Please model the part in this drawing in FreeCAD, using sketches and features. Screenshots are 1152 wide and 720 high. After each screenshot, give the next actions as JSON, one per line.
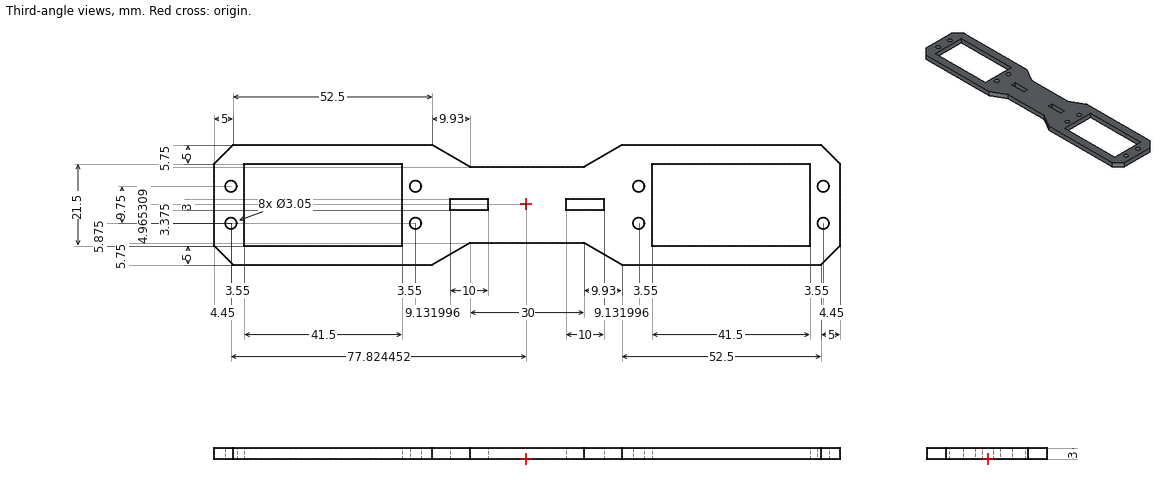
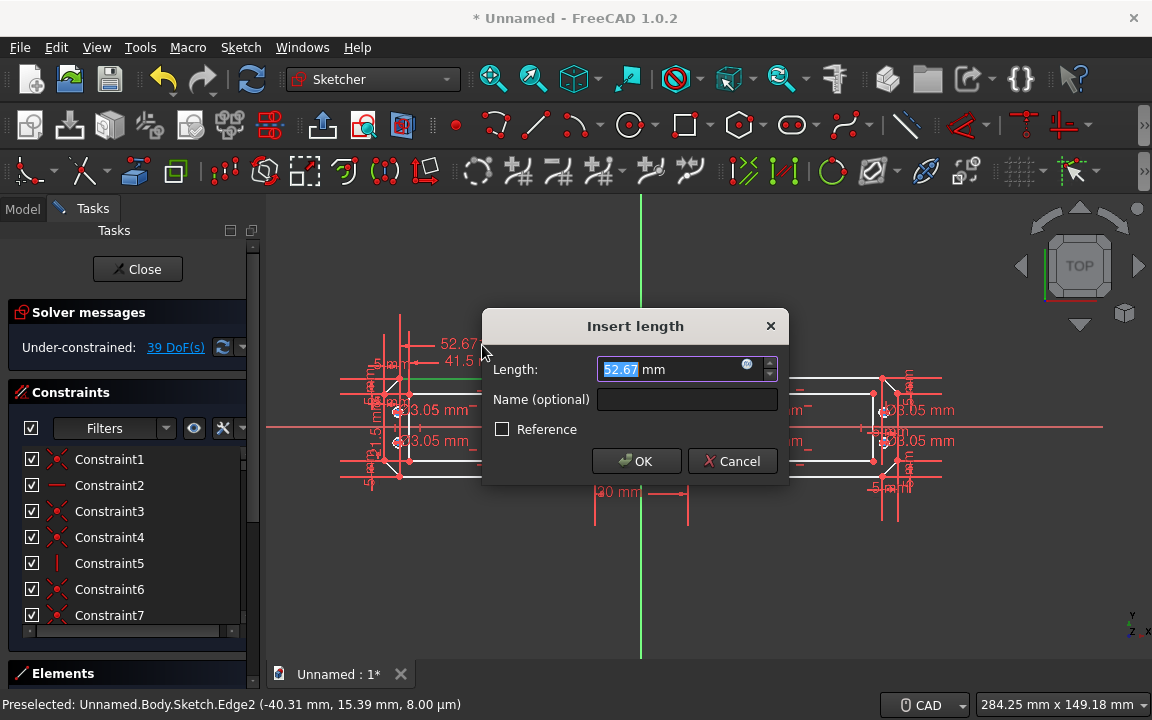
{"action": "type", "text": "52.5"}
{"action": "key", "text": "Return"}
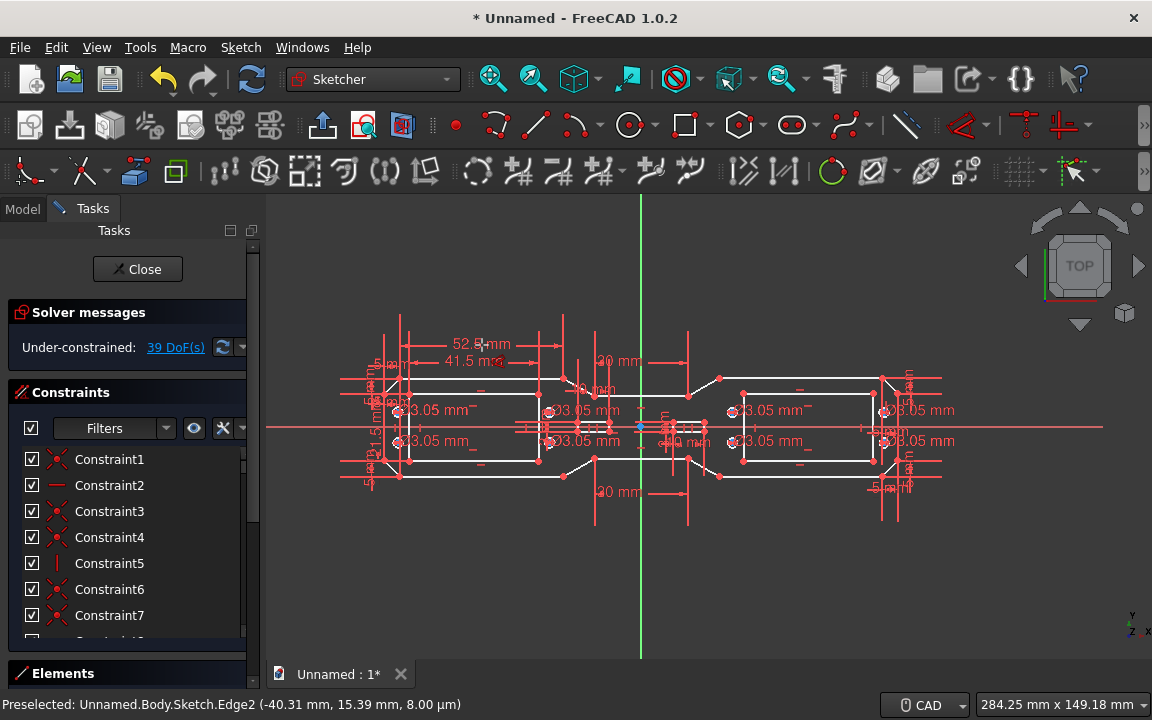
{"action": "scroll", "coordinate": [384, 414], "scroll_direction": "up", "scroll_amount": 3}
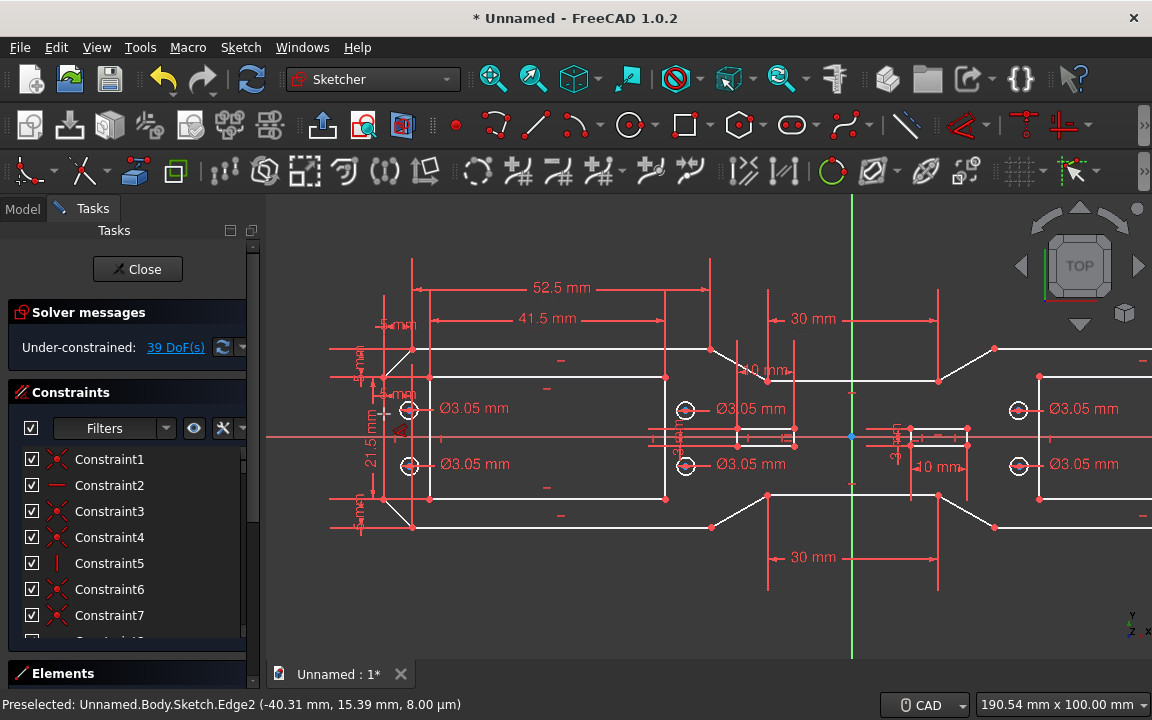
{"action": "left_click", "coordinate": [384, 414]}
{"action": "left_click", "coordinate": [350, 466]}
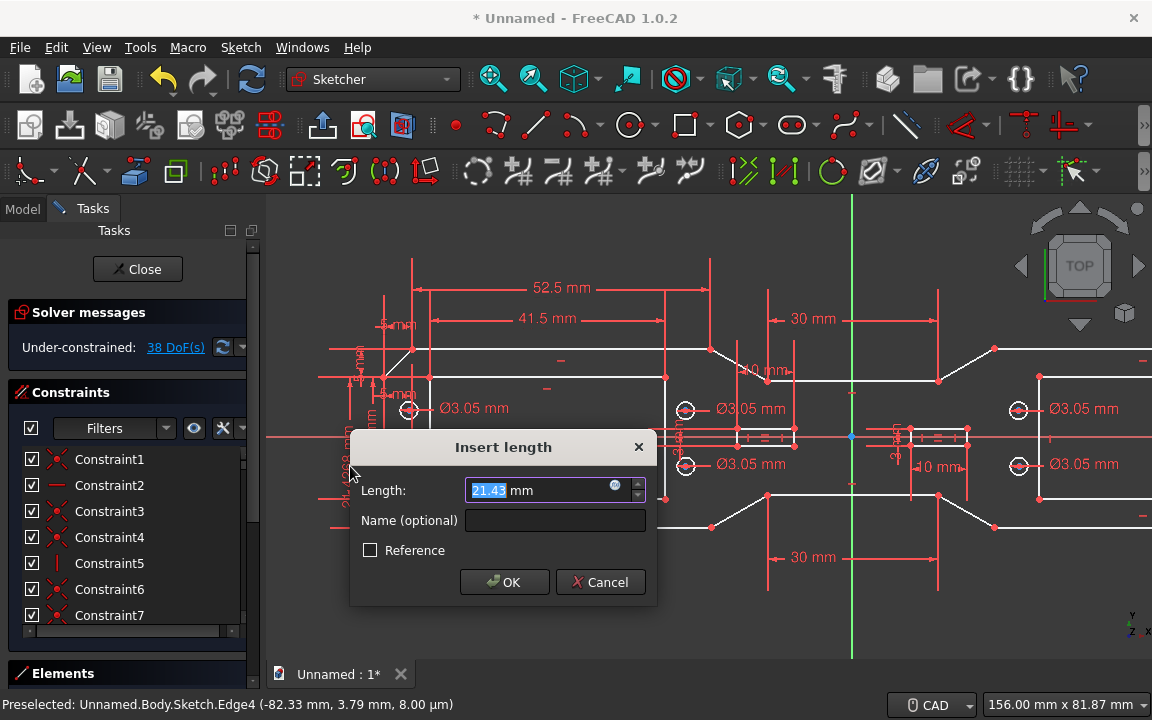
{"action": "type", "text": "21.5"}
{"action": "key", "text": "Return"}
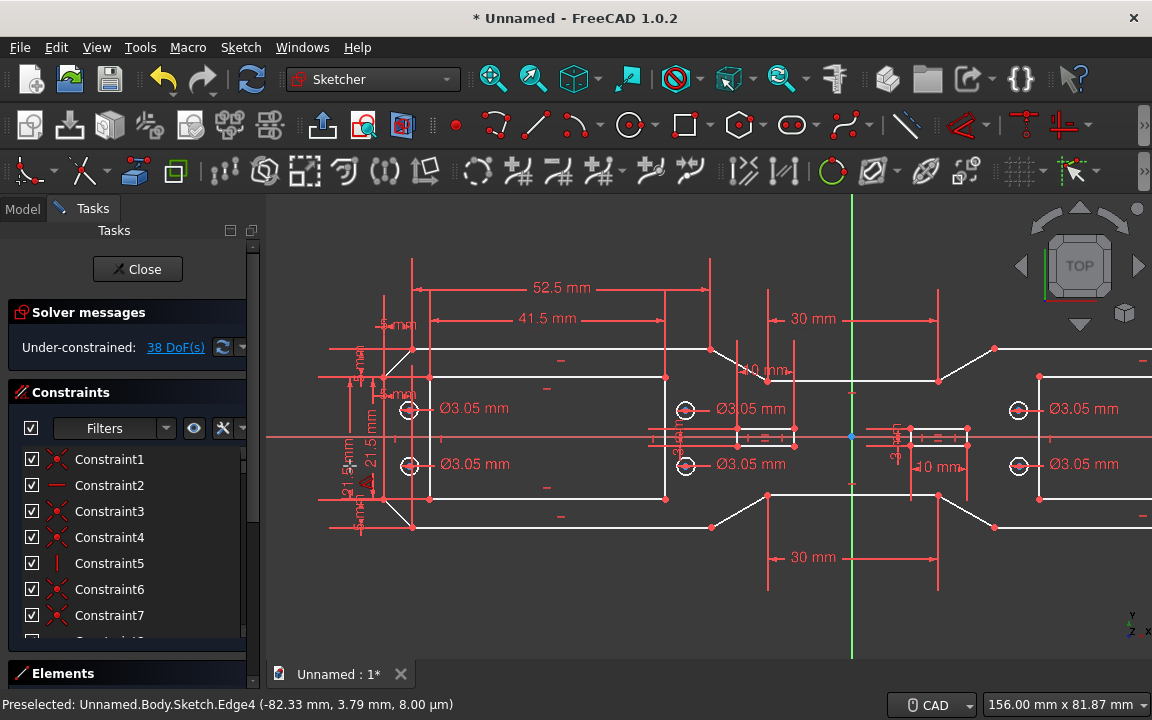
{"action": "left_click", "coordinate": [502, 528]}
{"action": "left_click", "coordinate": [562, 562]}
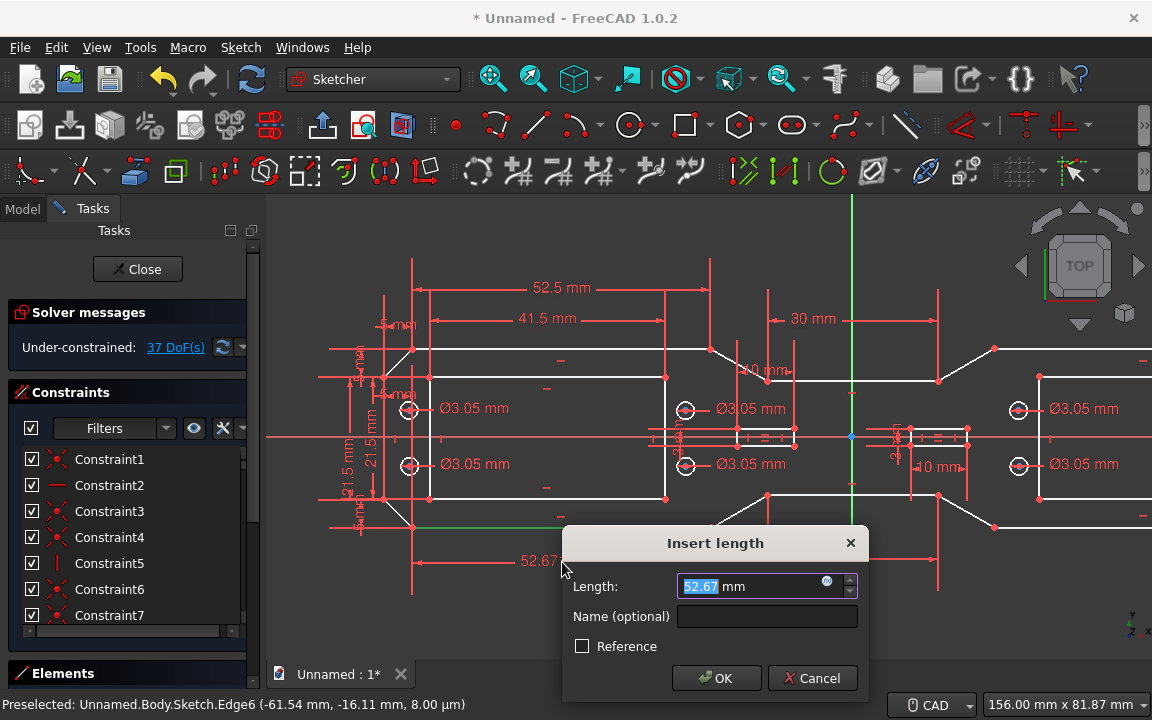
{"action": "type", "text": "52.5"}
{"action": "key", "text": "Return"}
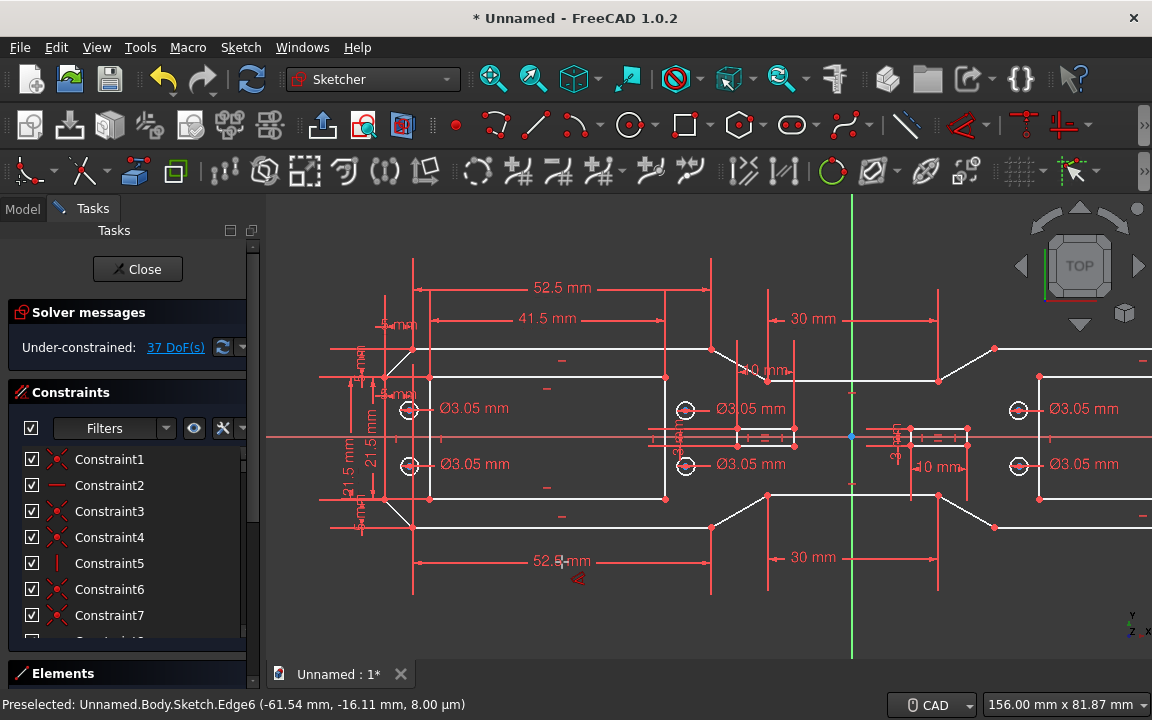
{"action": "scroll", "coordinate": [383, 414], "scroll_direction": "down", "scroll_amount": 3}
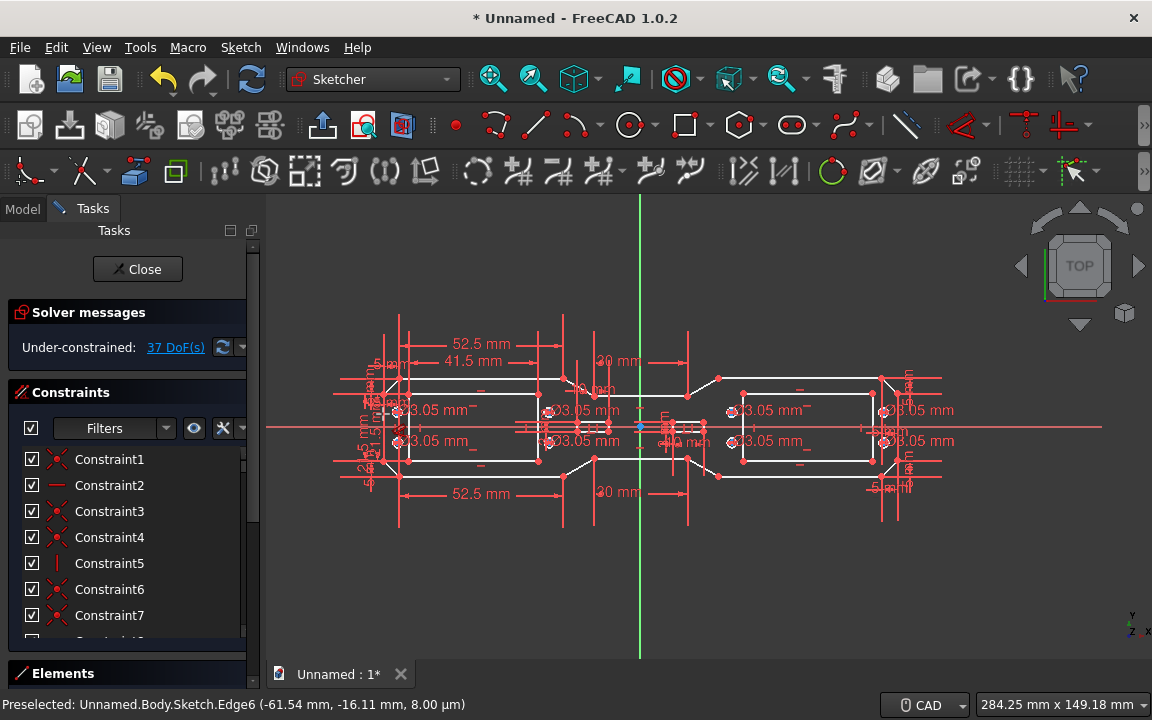
{"action": "left_click", "coordinate": [768, 477]}
{"action": "left_click", "coordinate": [800, 511]}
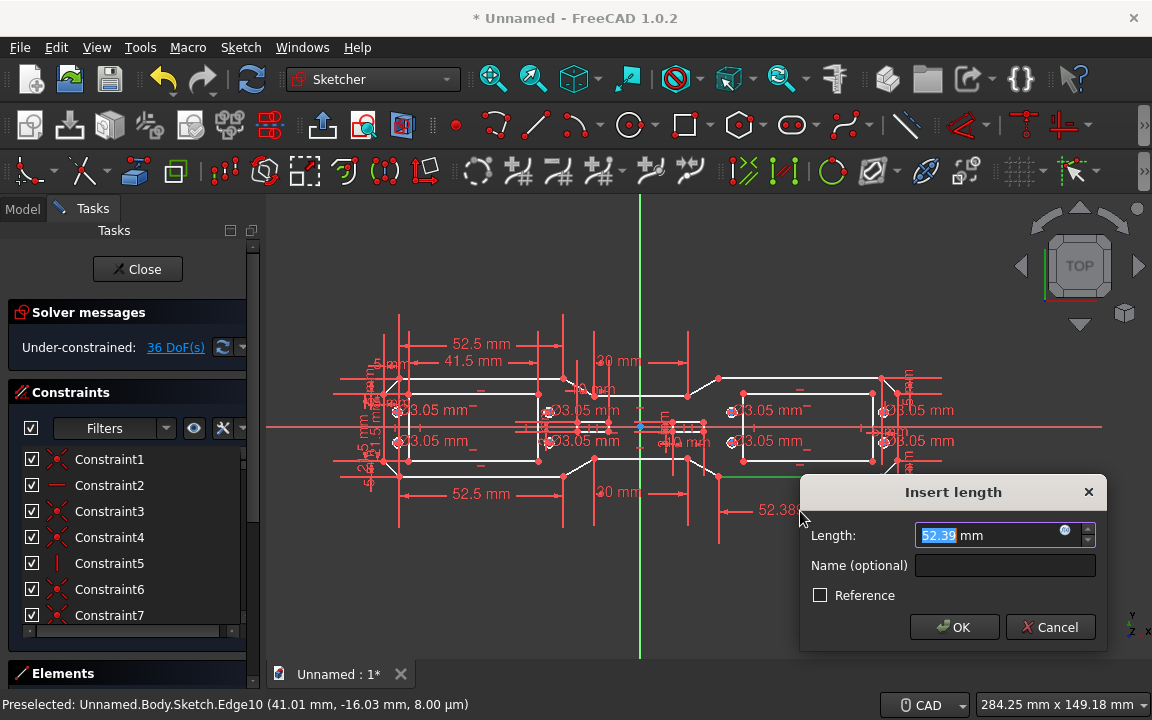
{"action": "type", "text": "52.5"}
{"action": "key", "text": "Return"}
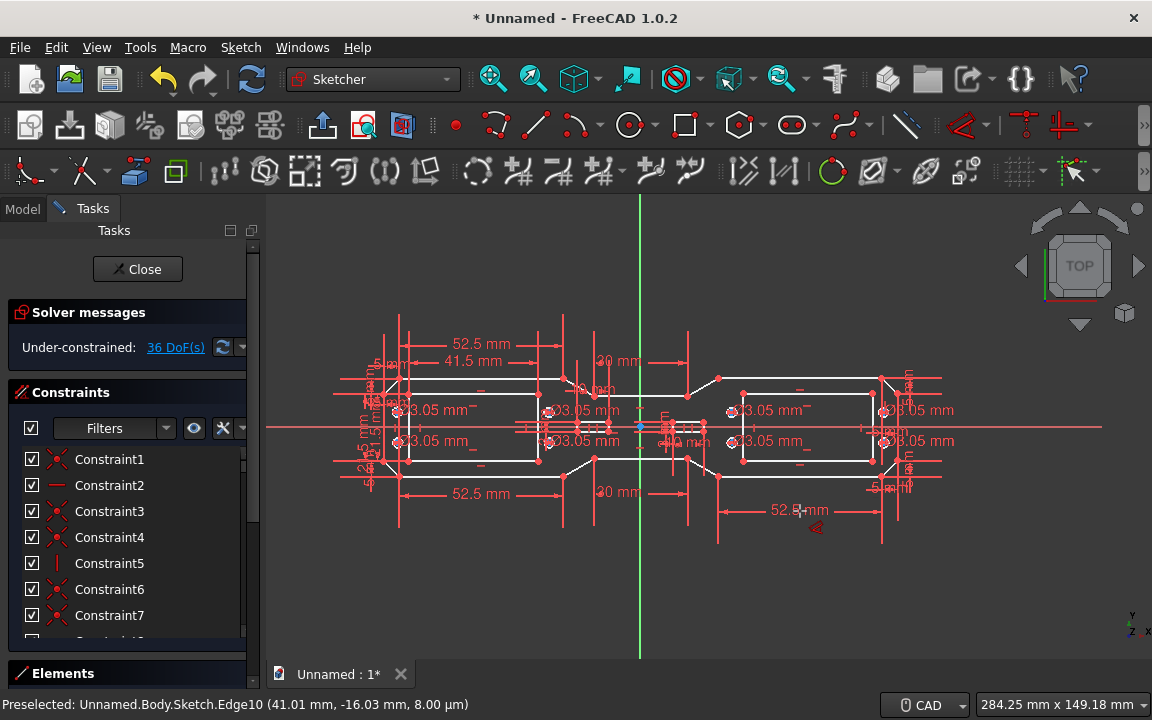
{"action": "scroll", "coordinate": [898, 441], "scroll_direction": "up", "scroll_amount": 3}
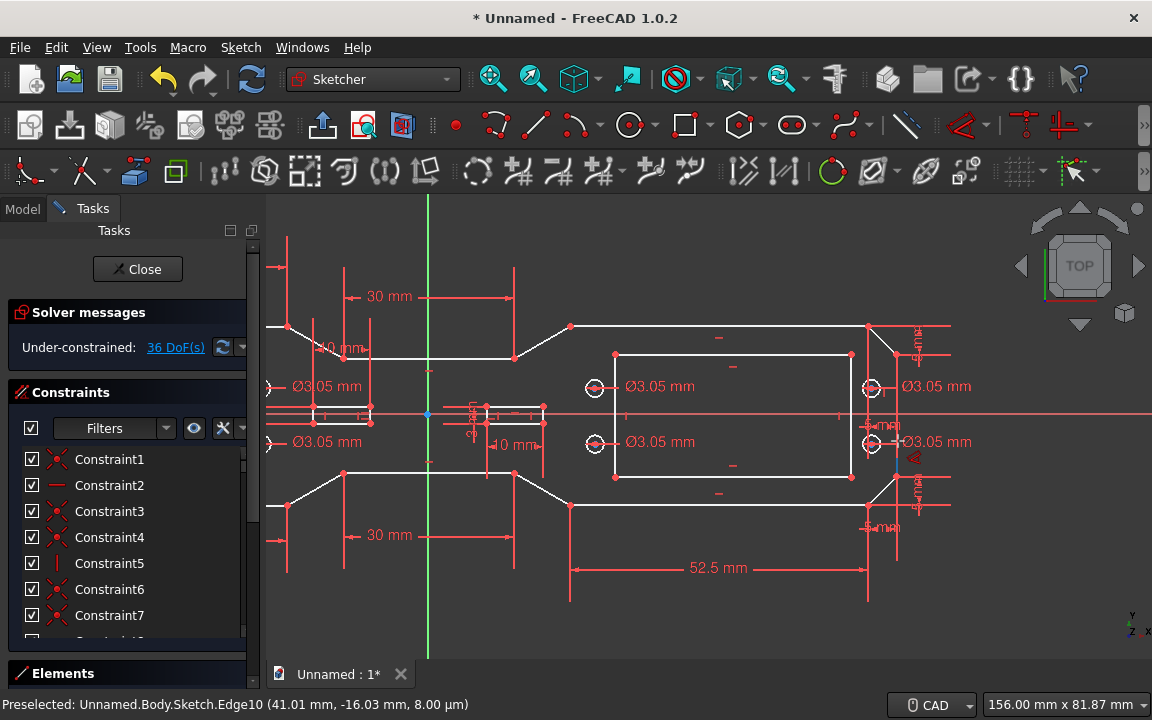
{"action": "left_click", "coordinate": [897, 440]}
{"action": "left_click", "coordinate": [931, 388]}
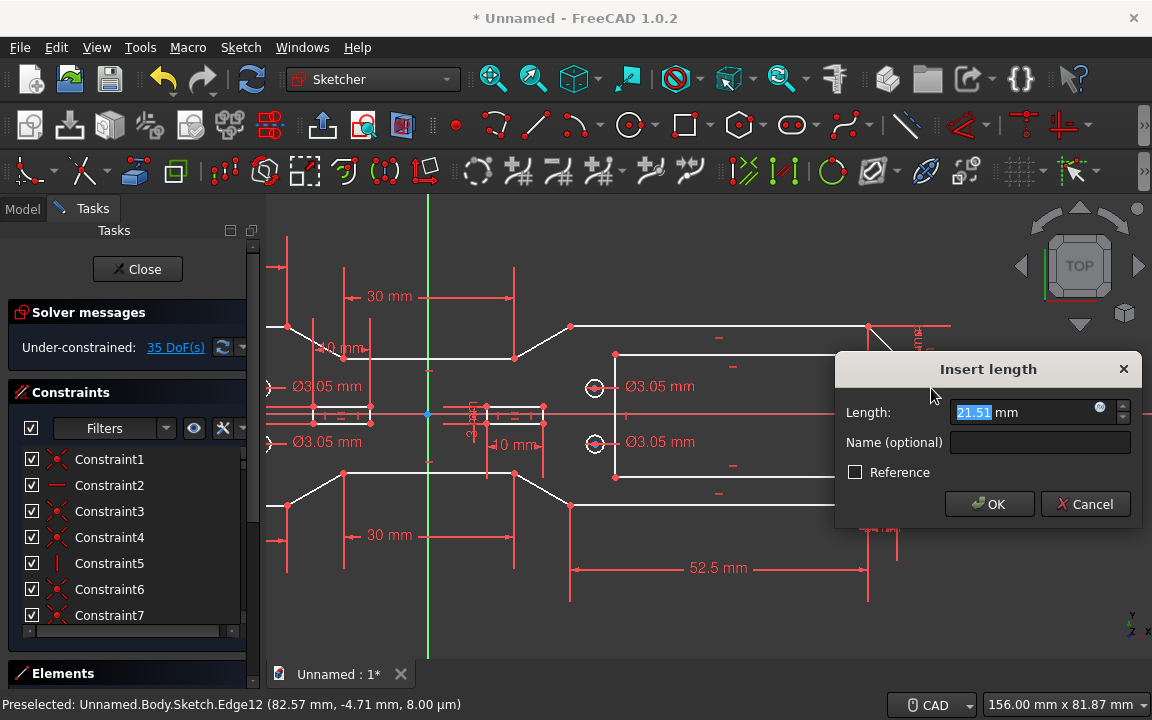
{"action": "type", "text": "21.5"}
{"action": "key", "text": "Return"}